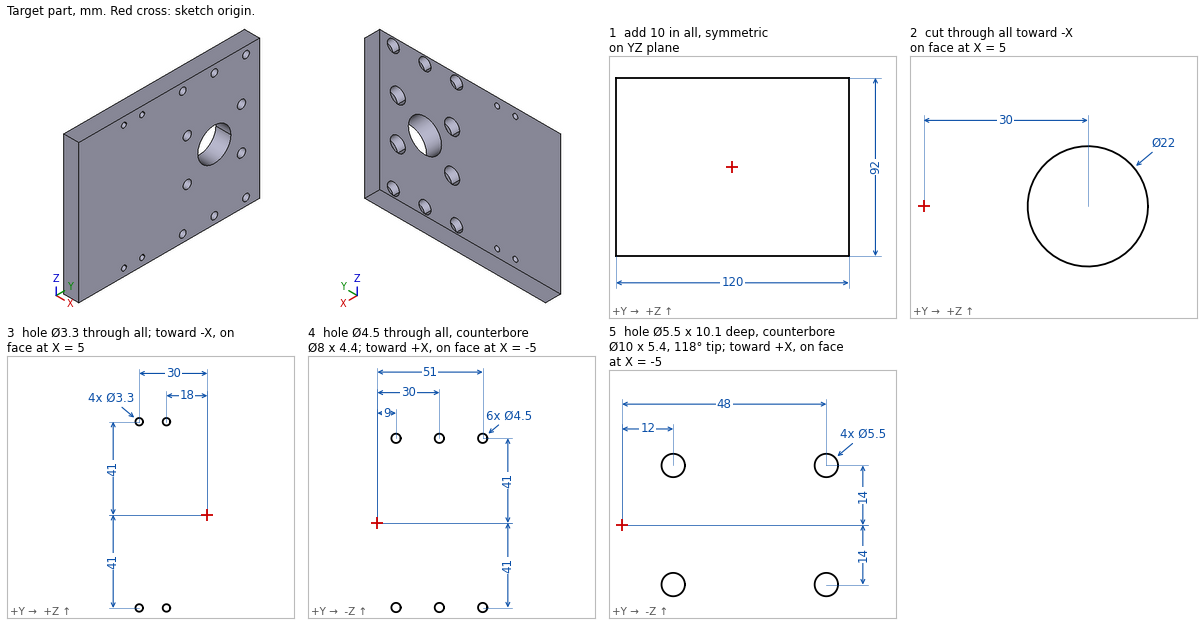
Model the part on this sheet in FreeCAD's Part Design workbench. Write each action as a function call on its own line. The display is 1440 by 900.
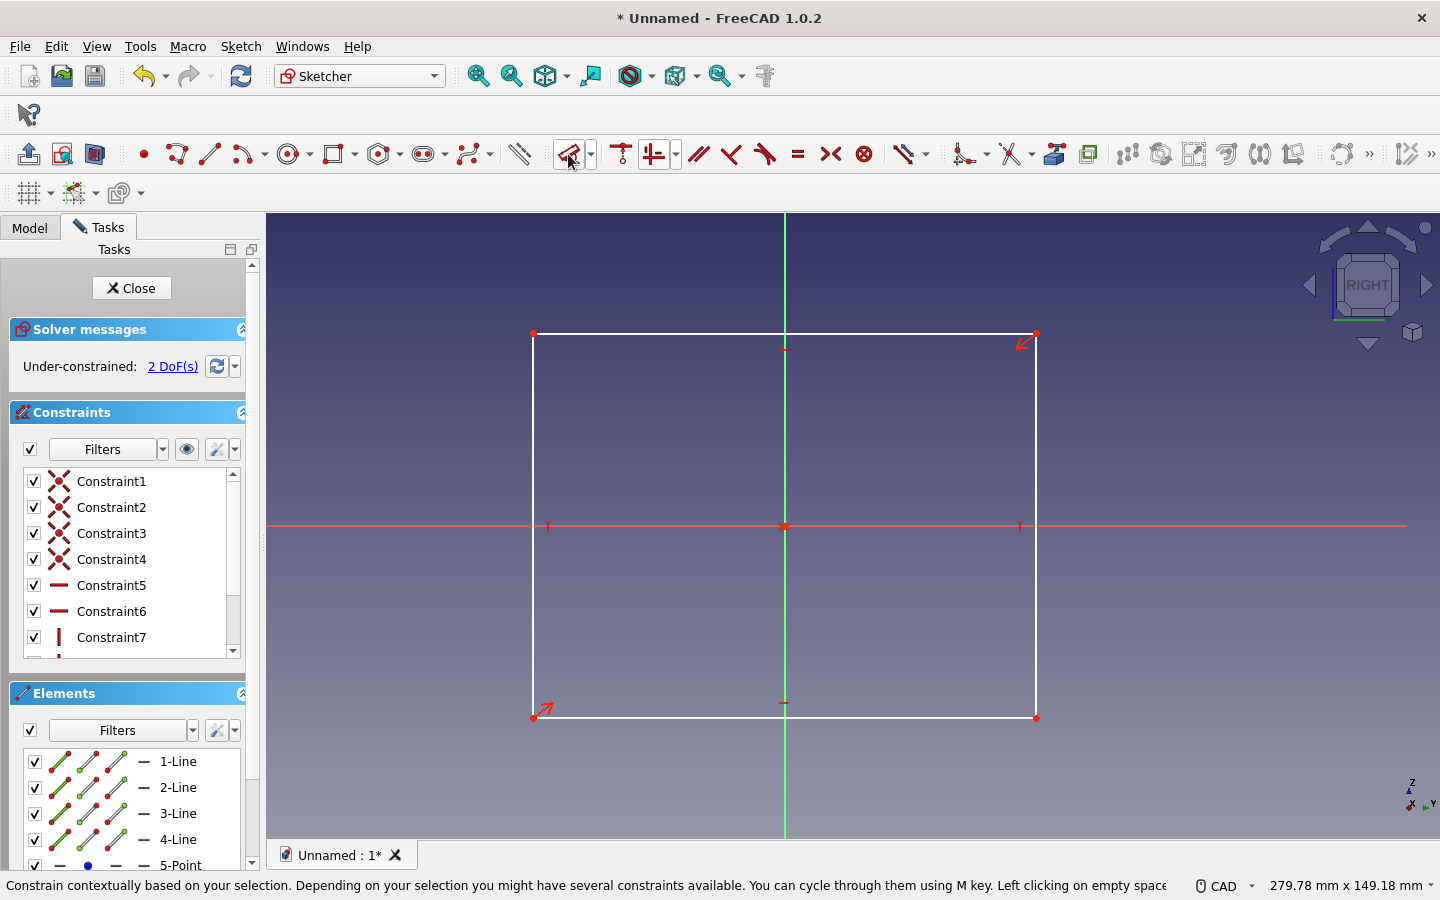
click(1036, 603)
click(1070, 438)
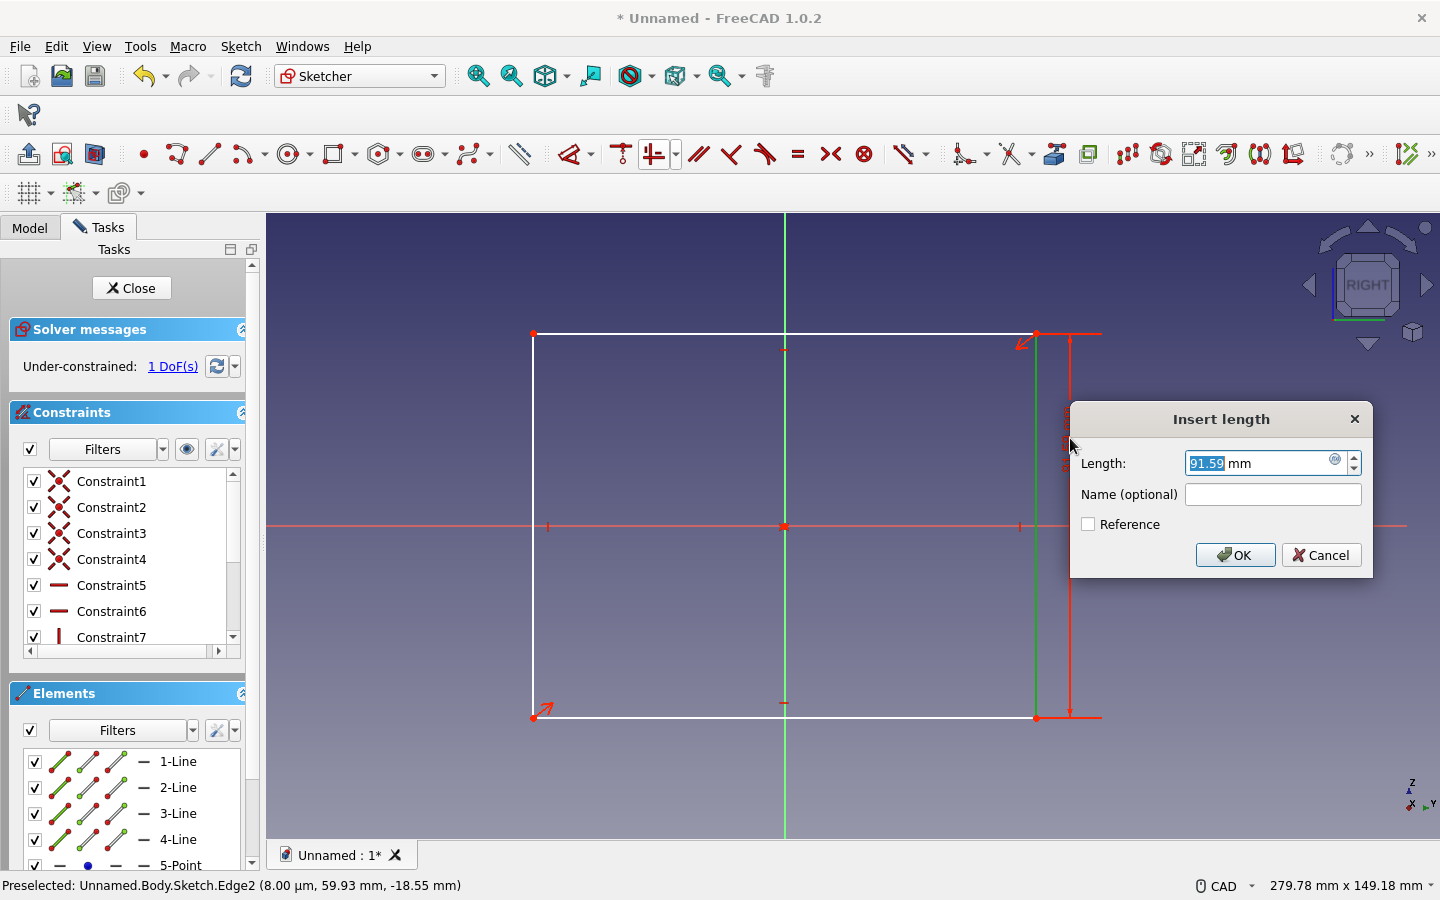
text(92)
key(Return)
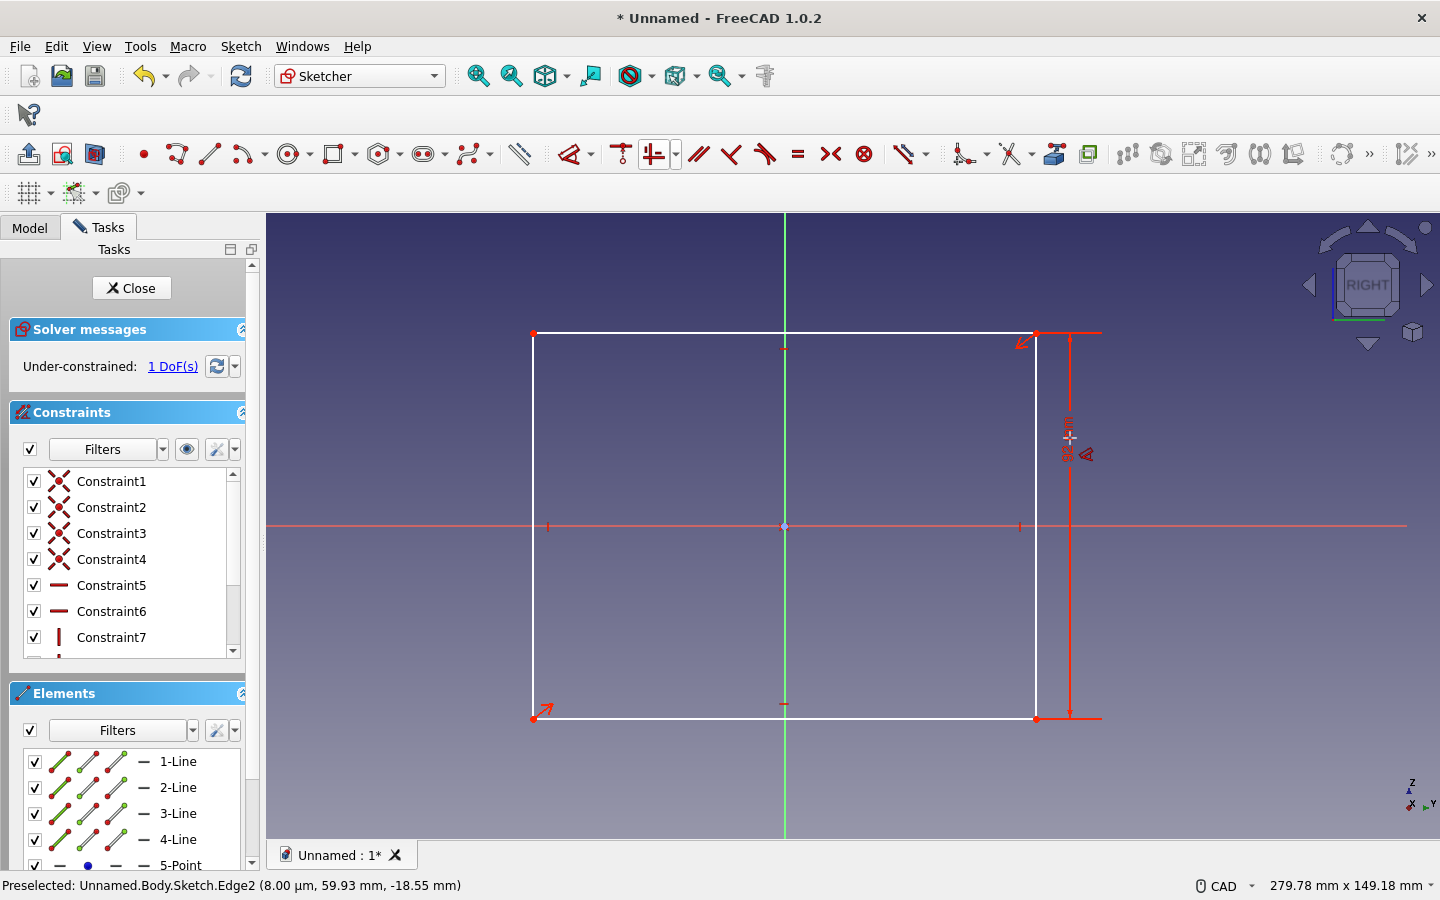
click(684, 719)
click(669, 753)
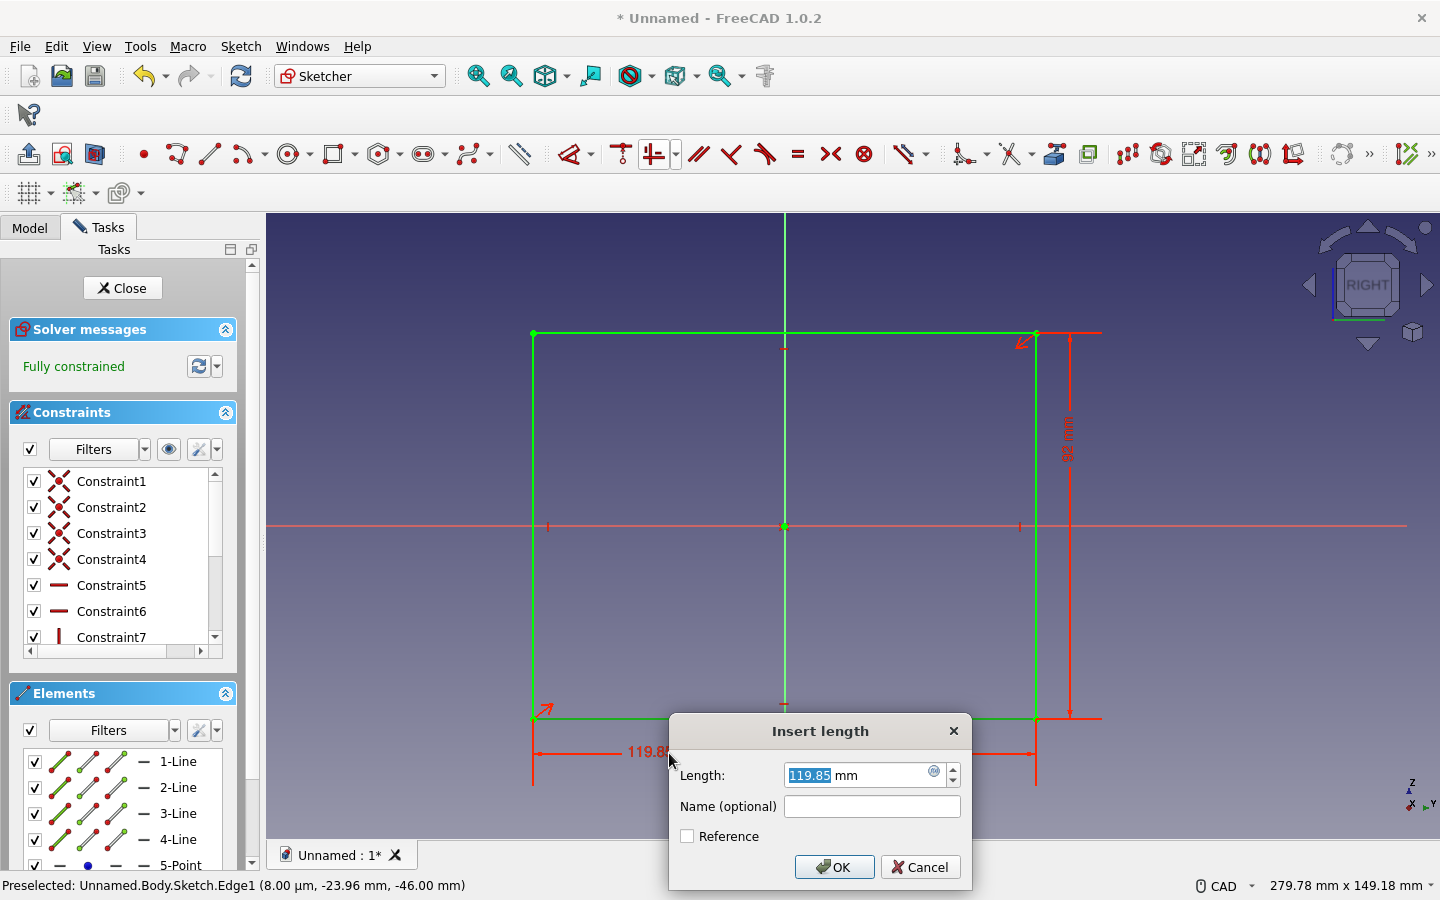
text(120)
key(Return)
key(Escape)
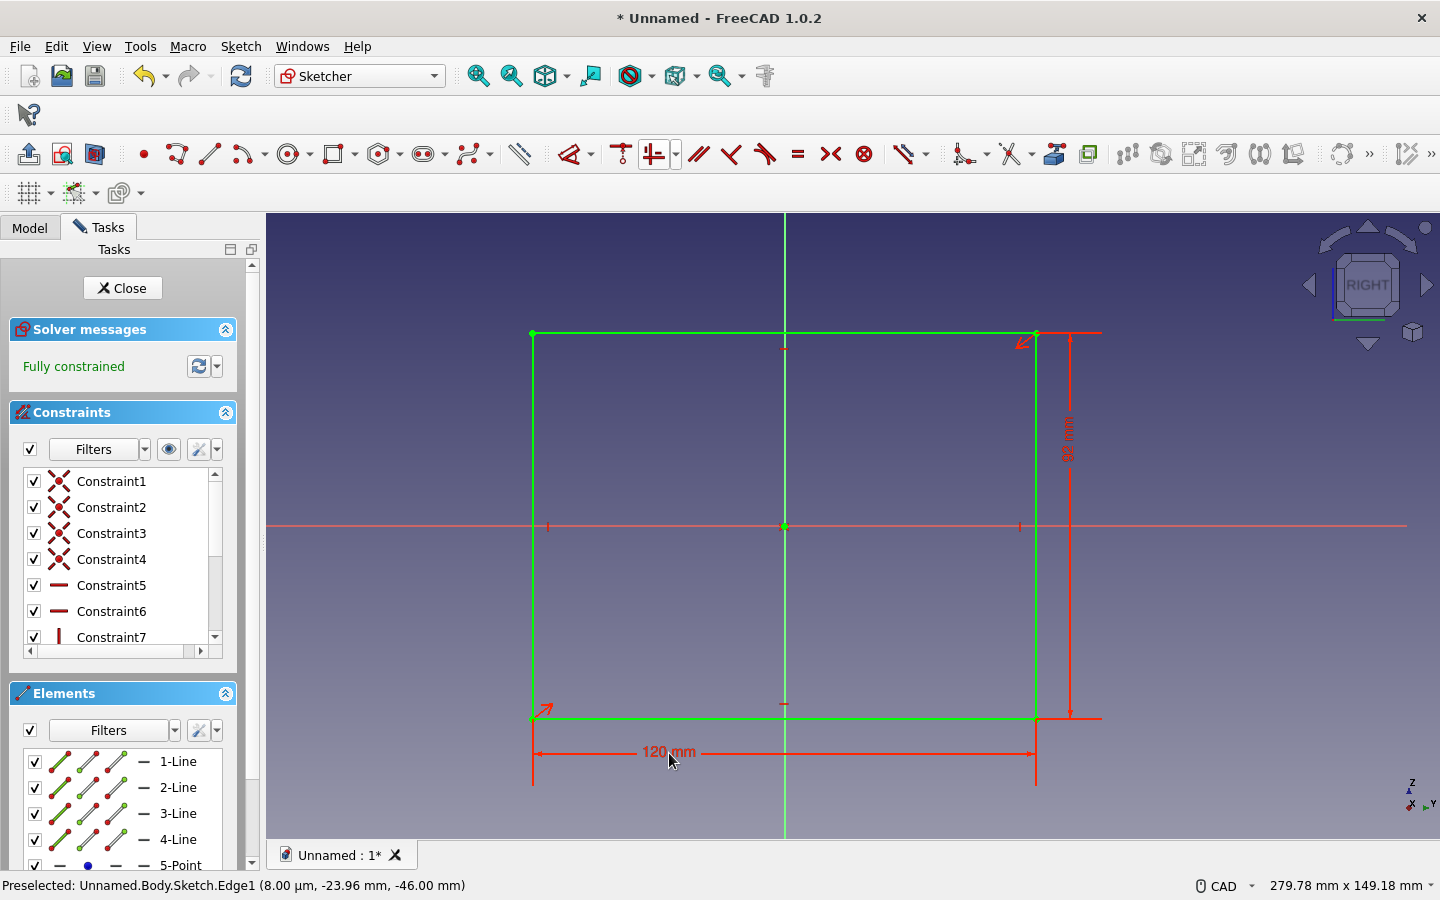
click(123, 288)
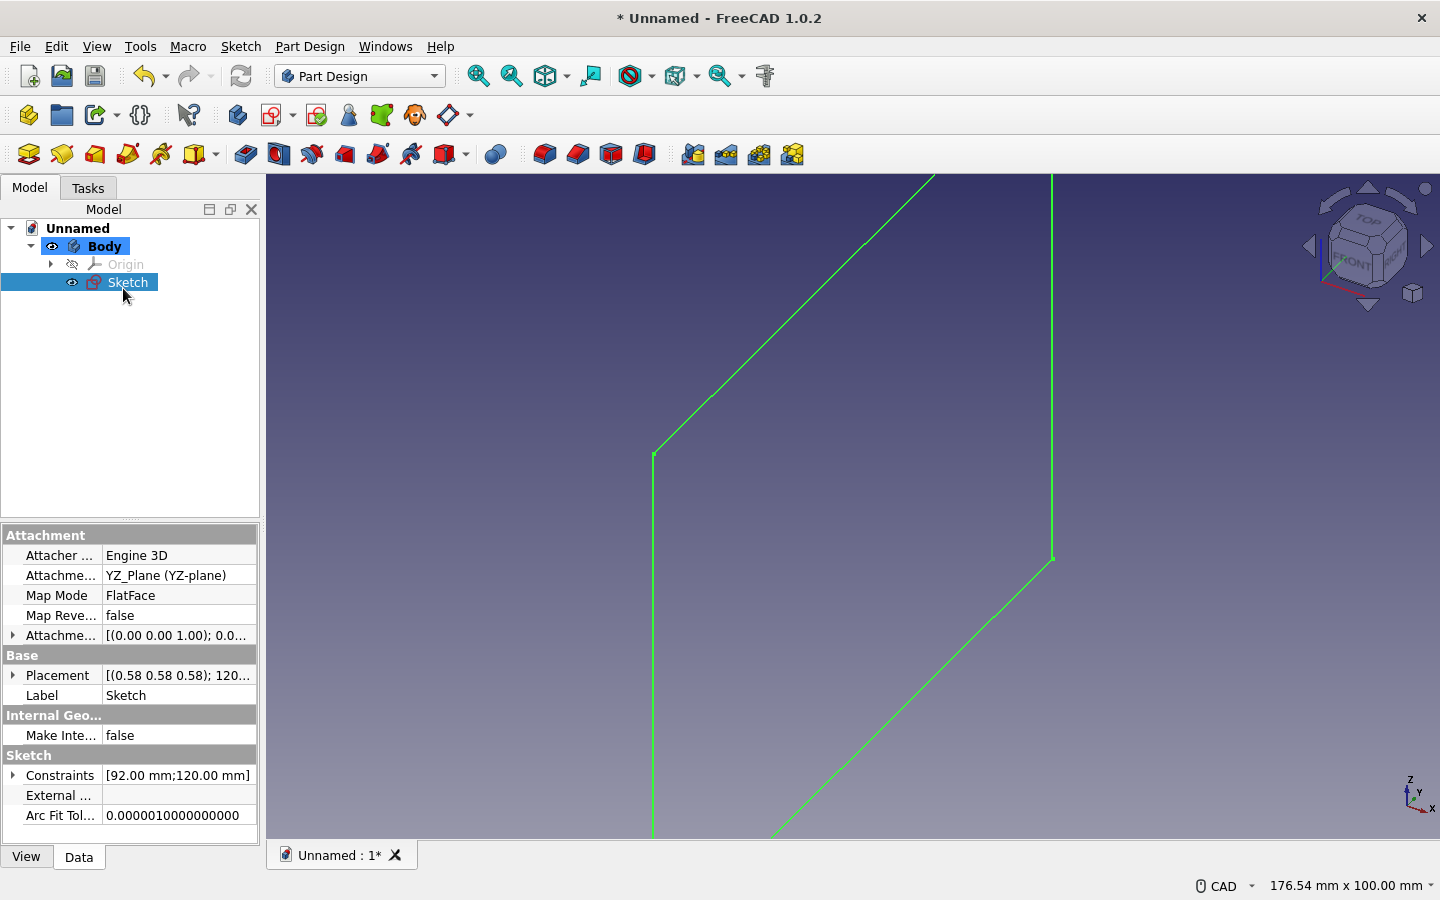
click(29, 154)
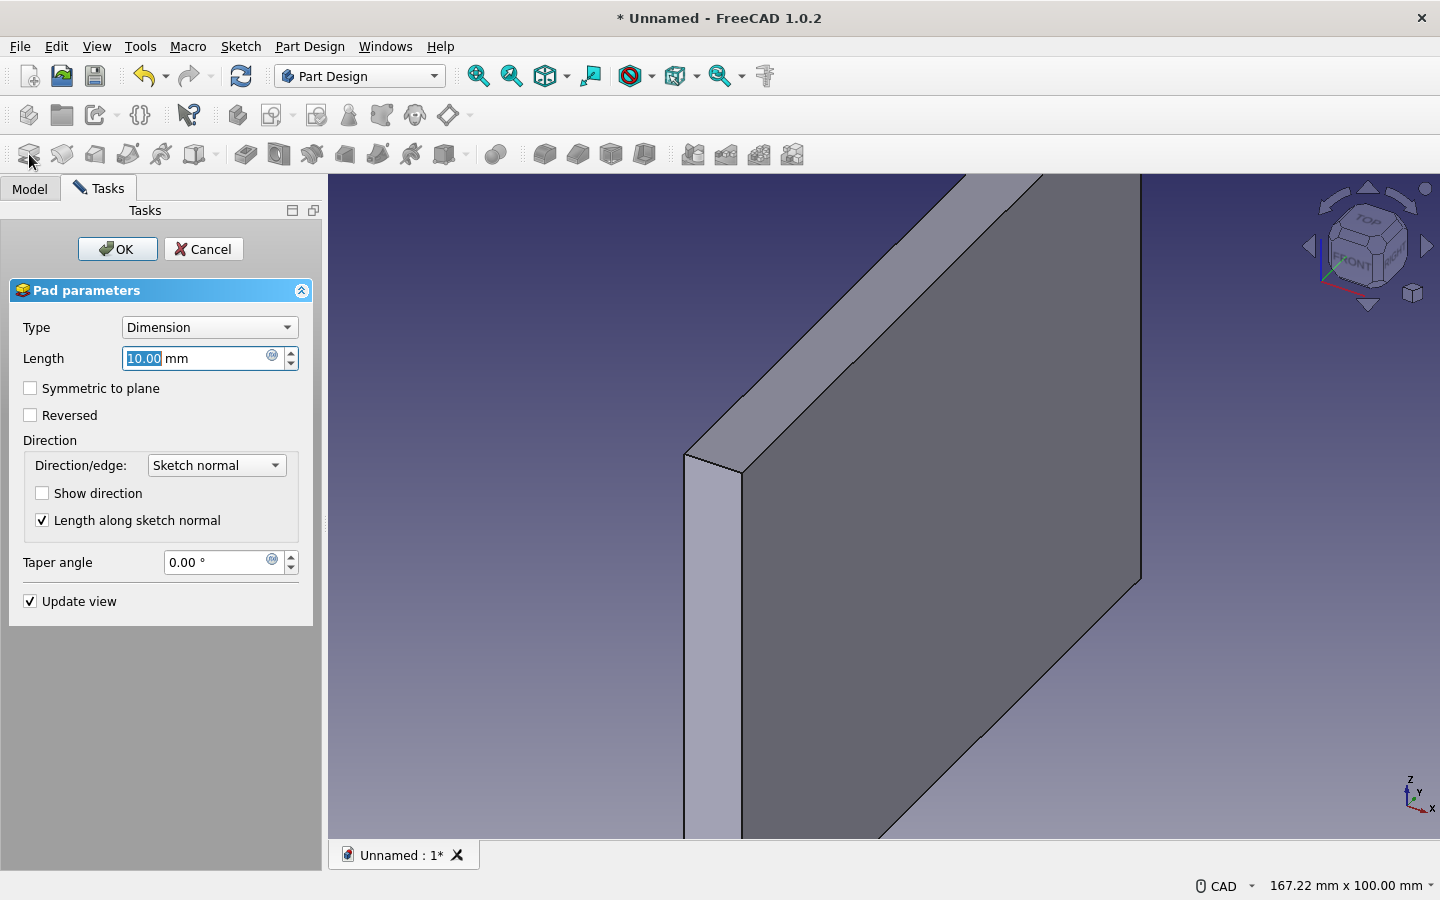
text(10)
key(Tab)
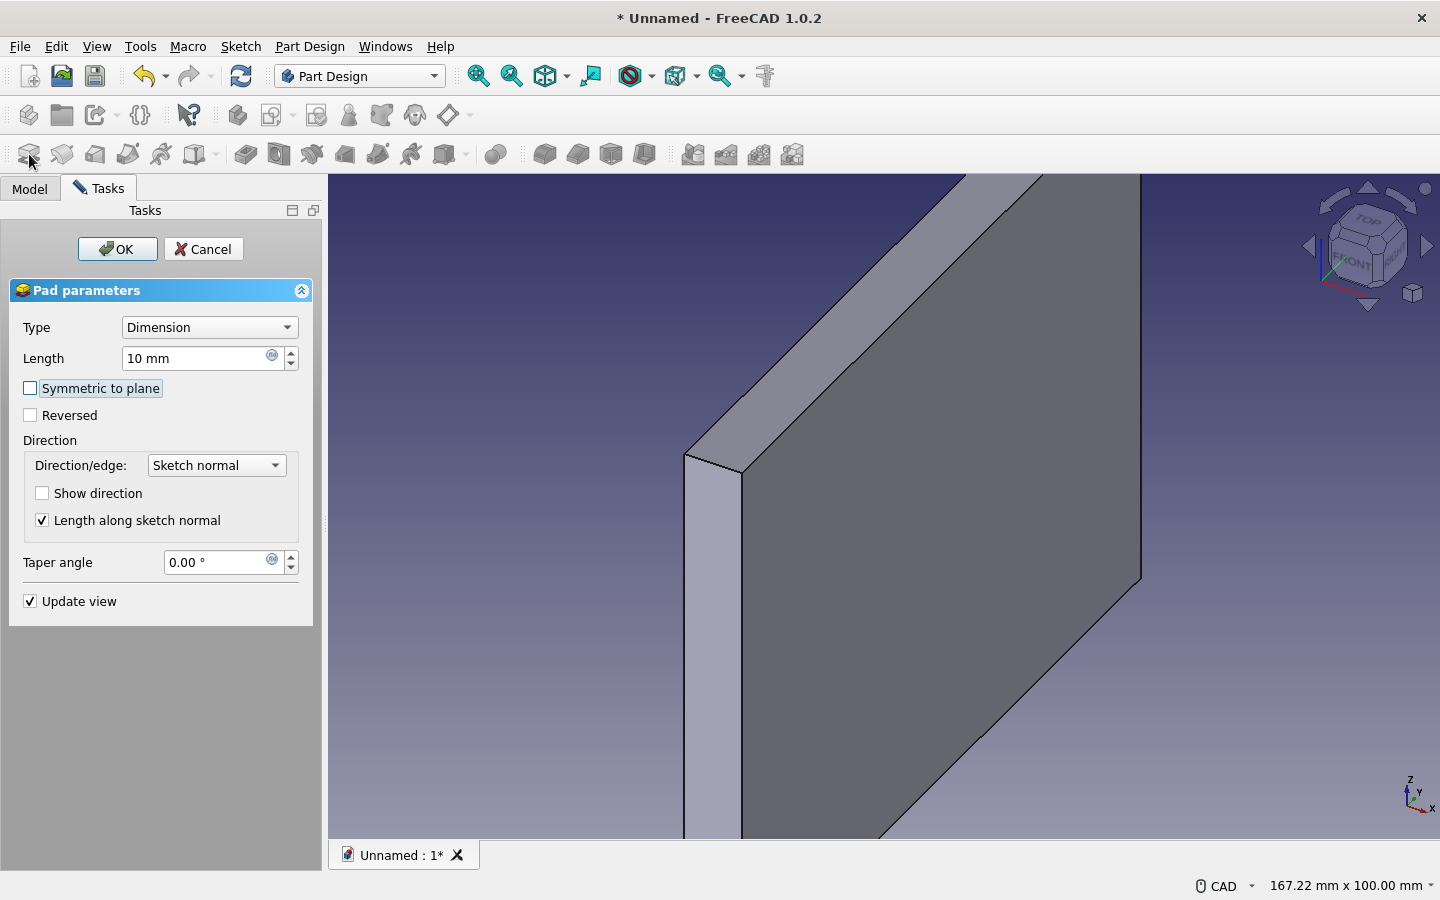
click(31, 388)